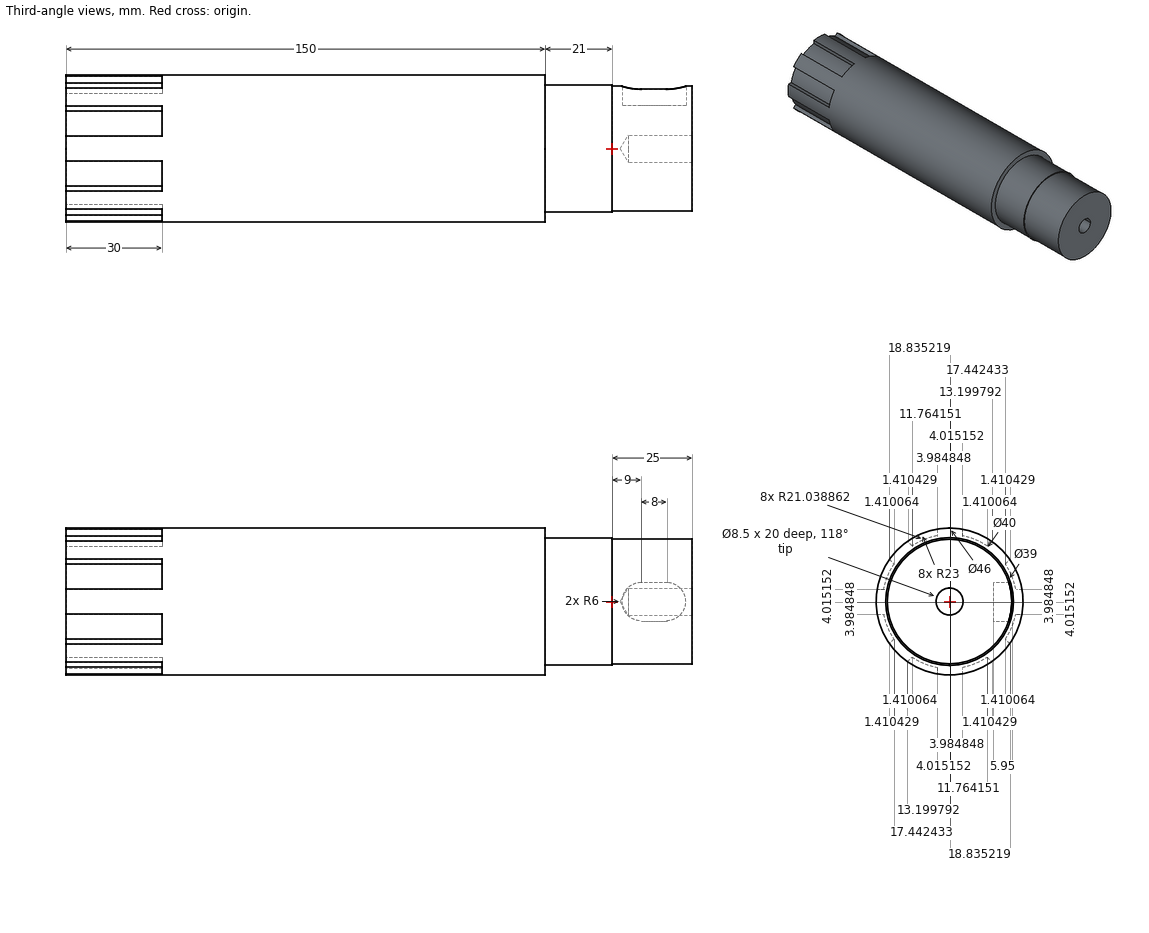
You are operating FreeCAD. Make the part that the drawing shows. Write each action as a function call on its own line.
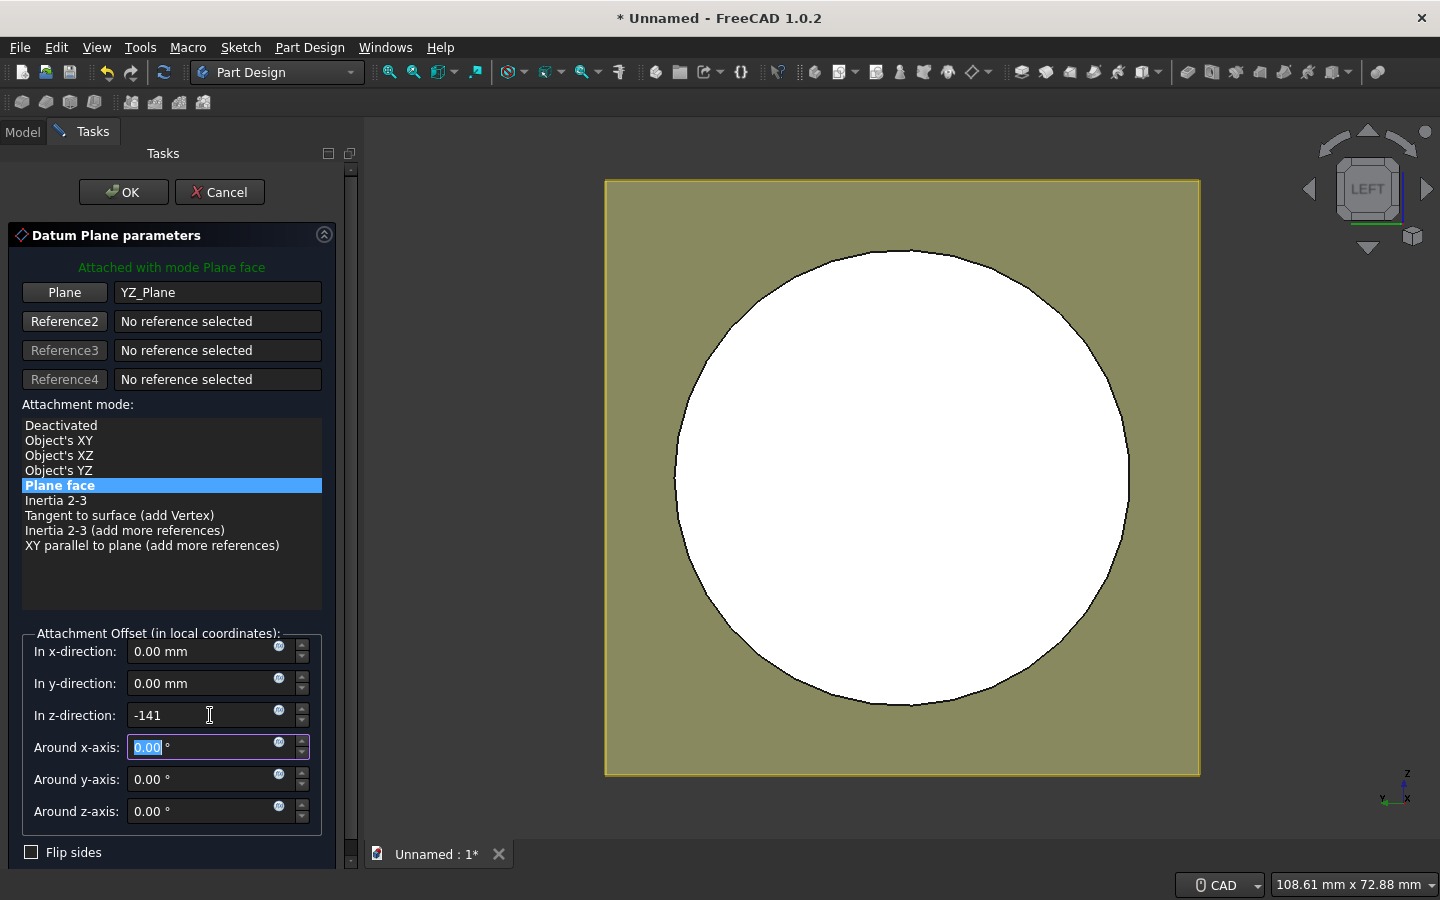
click(124, 192)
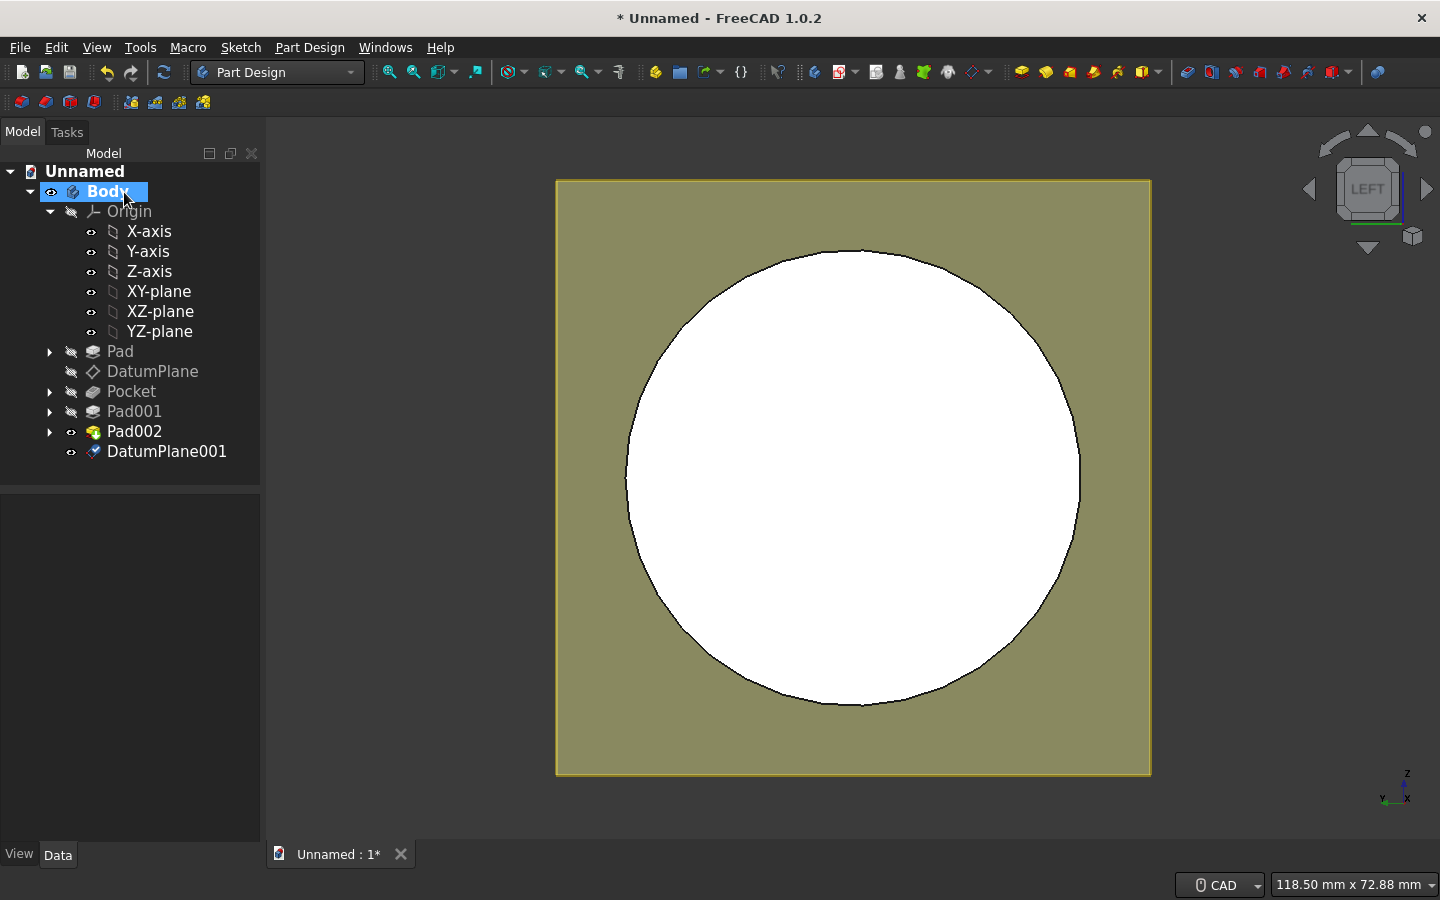
click(116, 452)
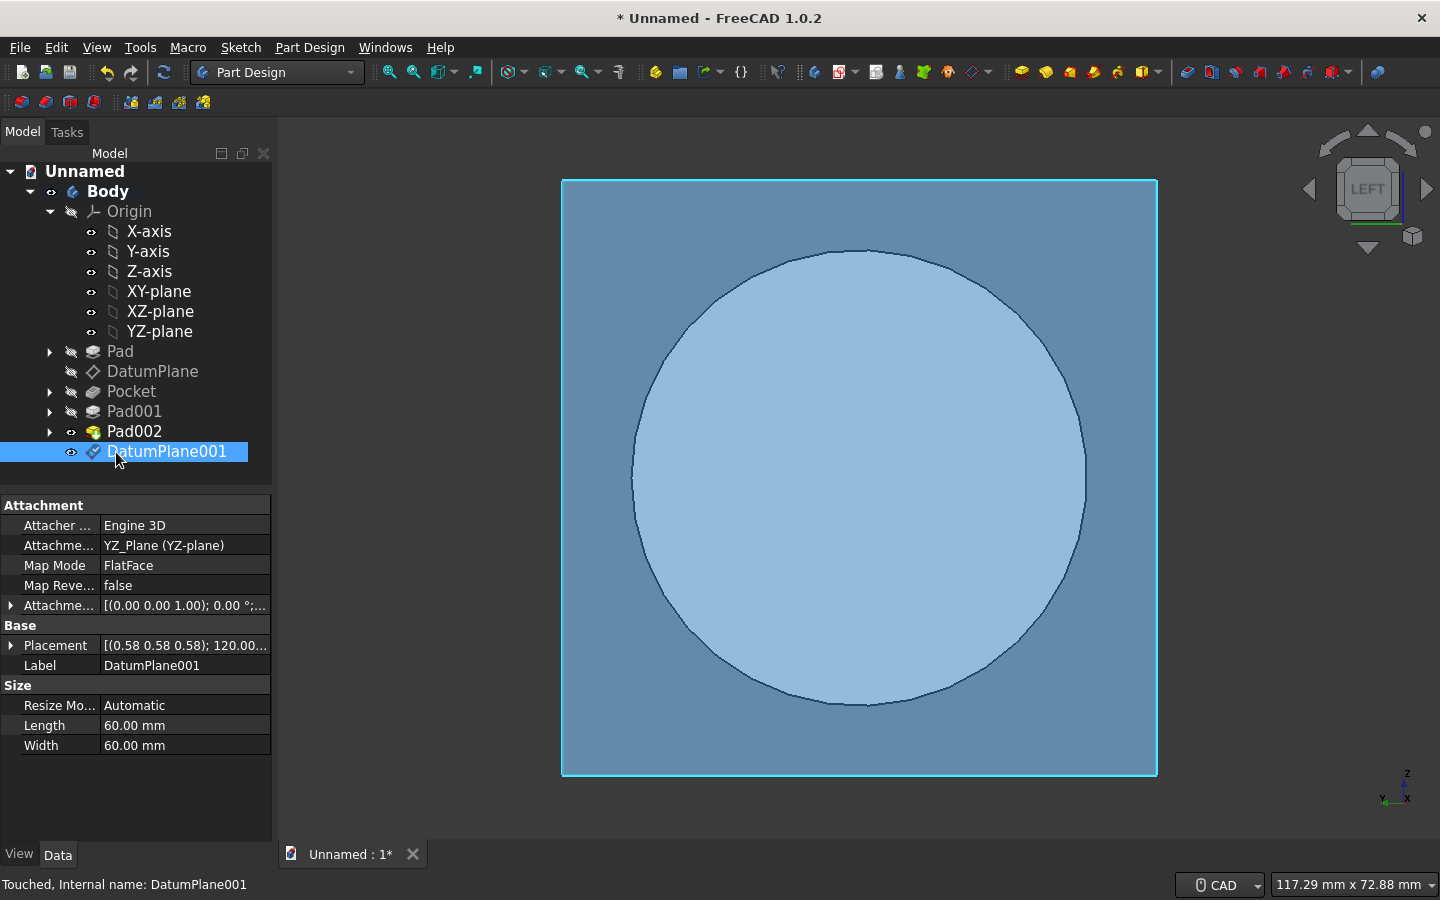
click(840, 72)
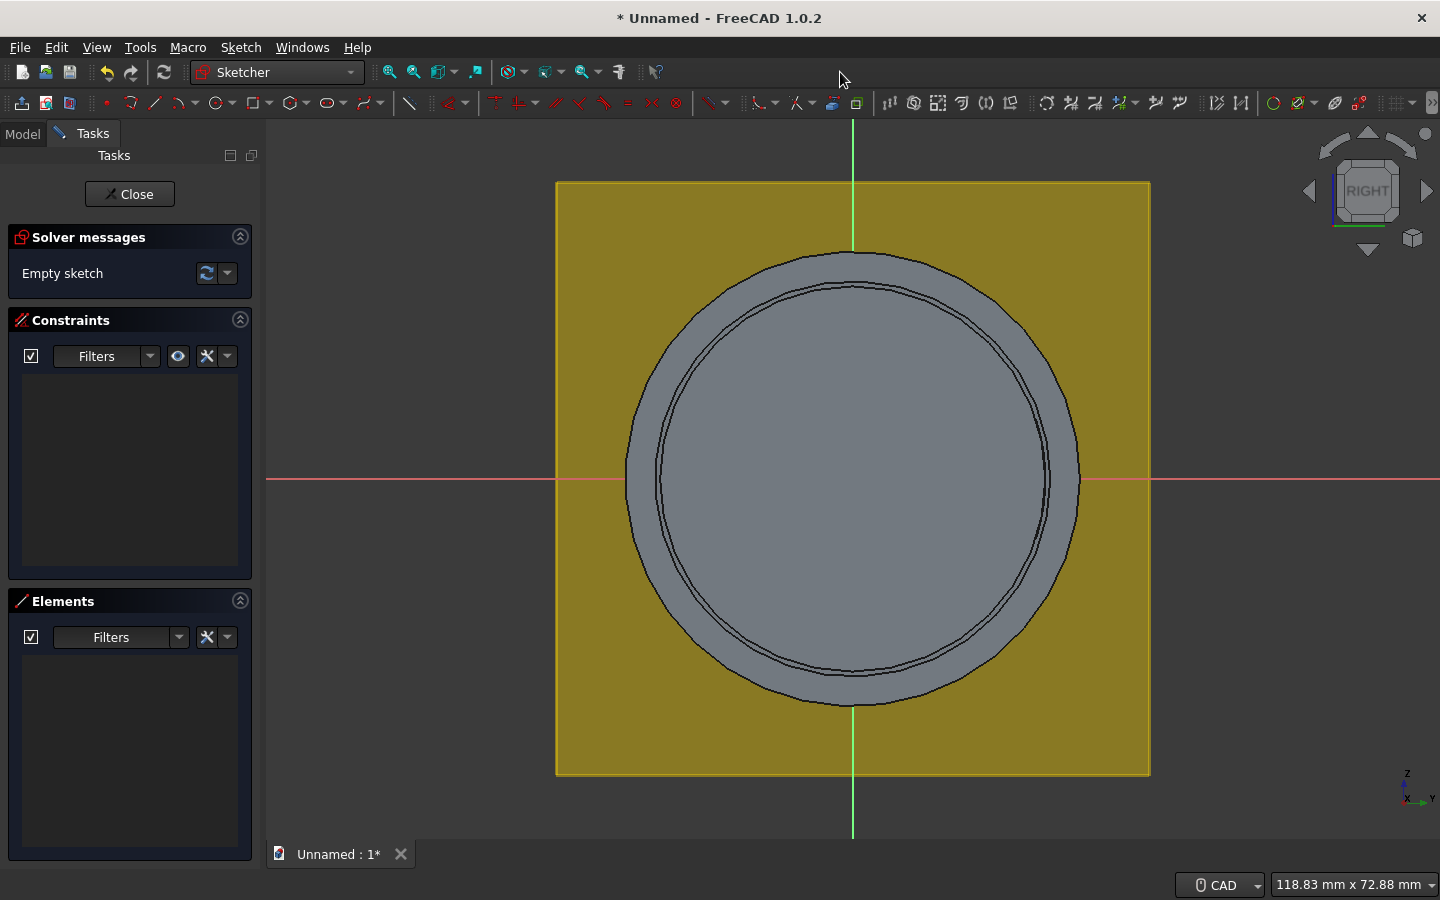
click(70, 104)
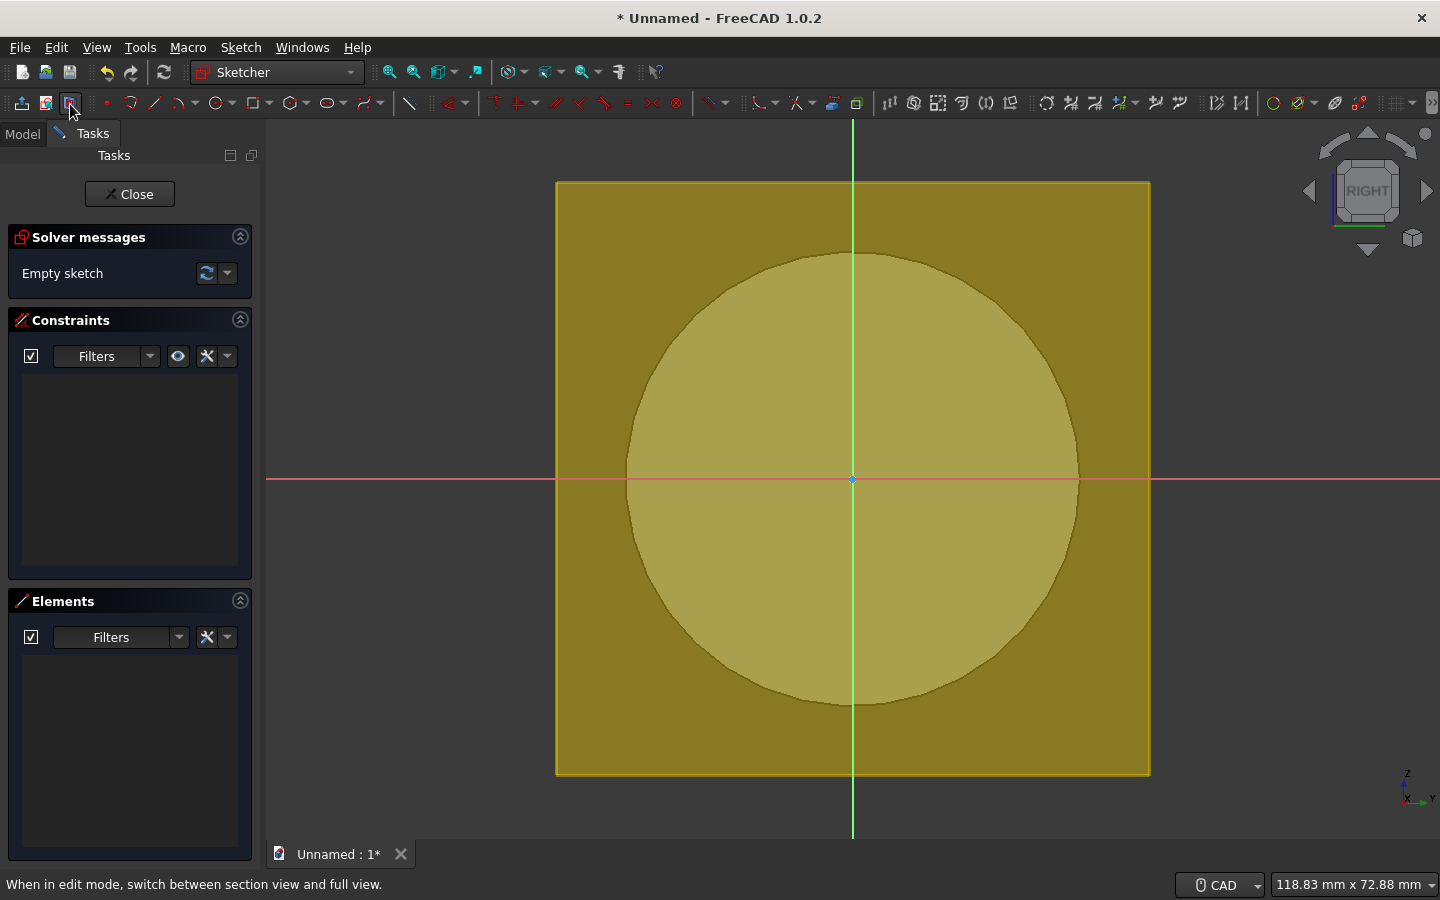
click(156, 104)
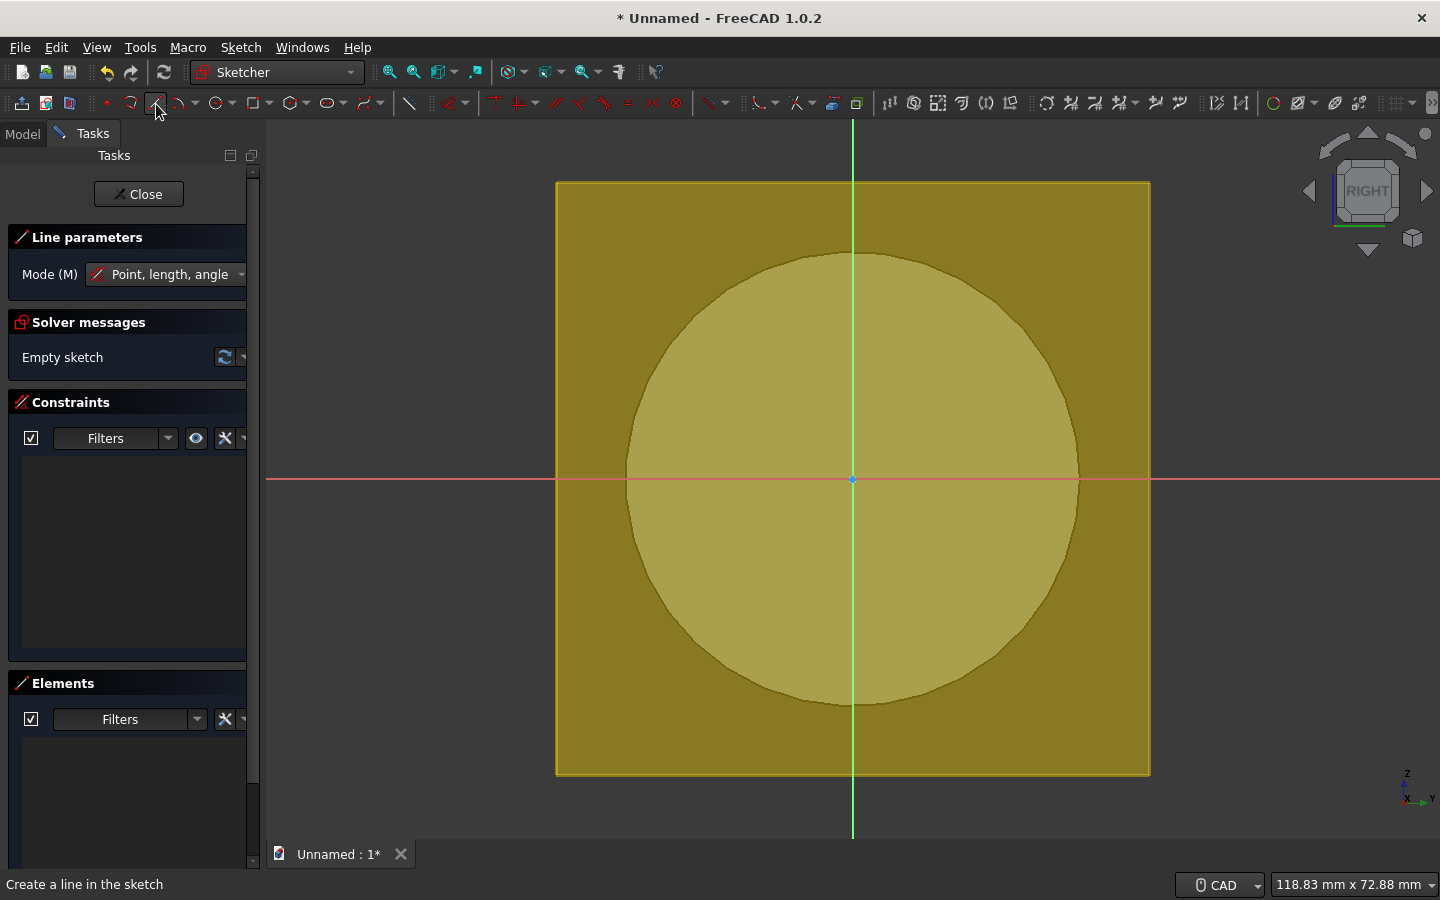
click(813, 255)
click(813, 275)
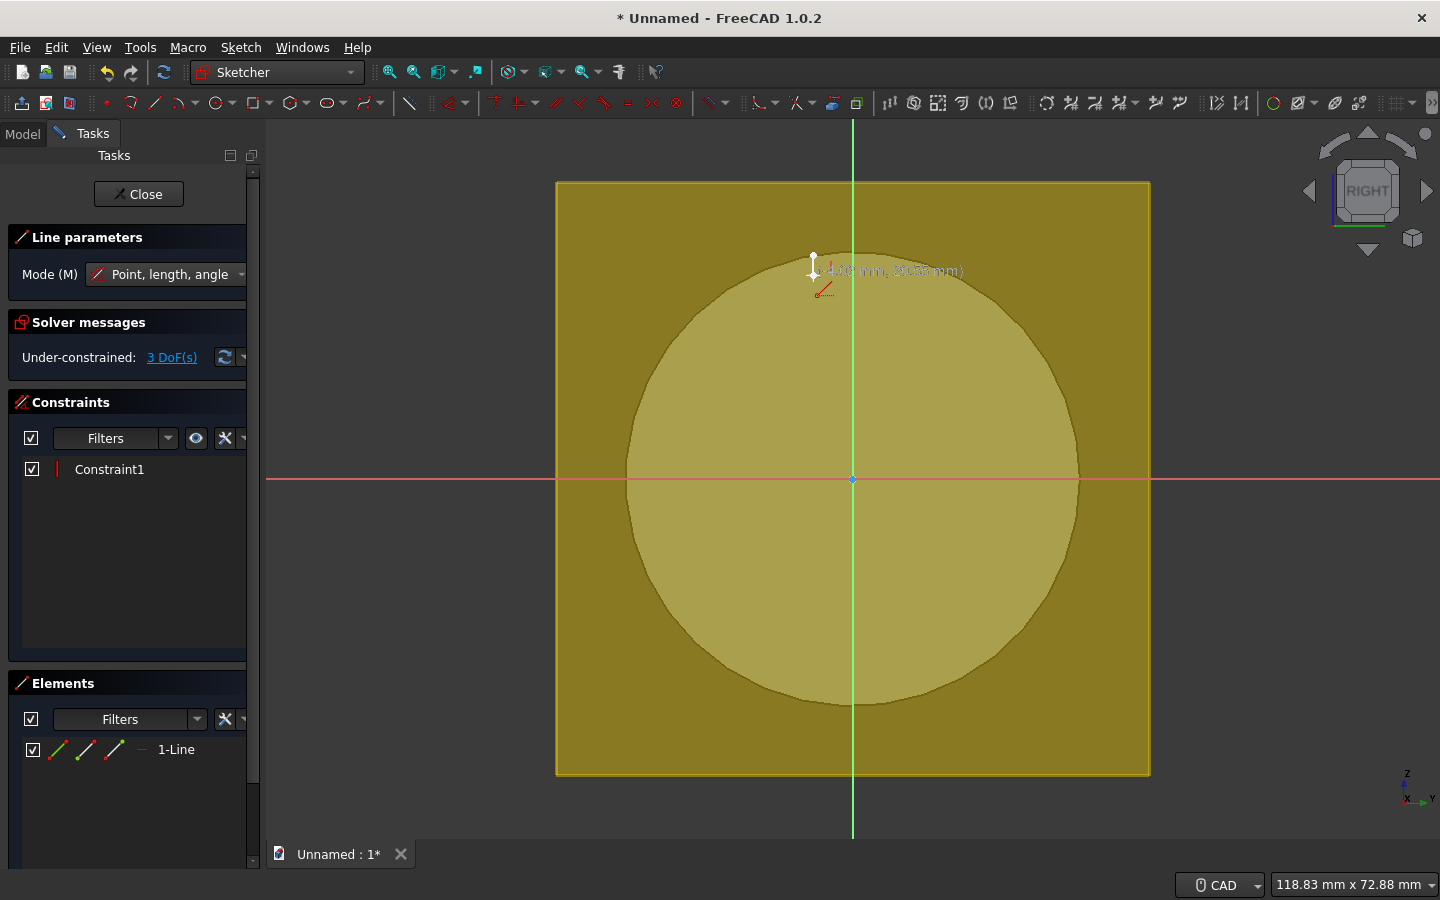
click(736, 307)
click(723, 293)